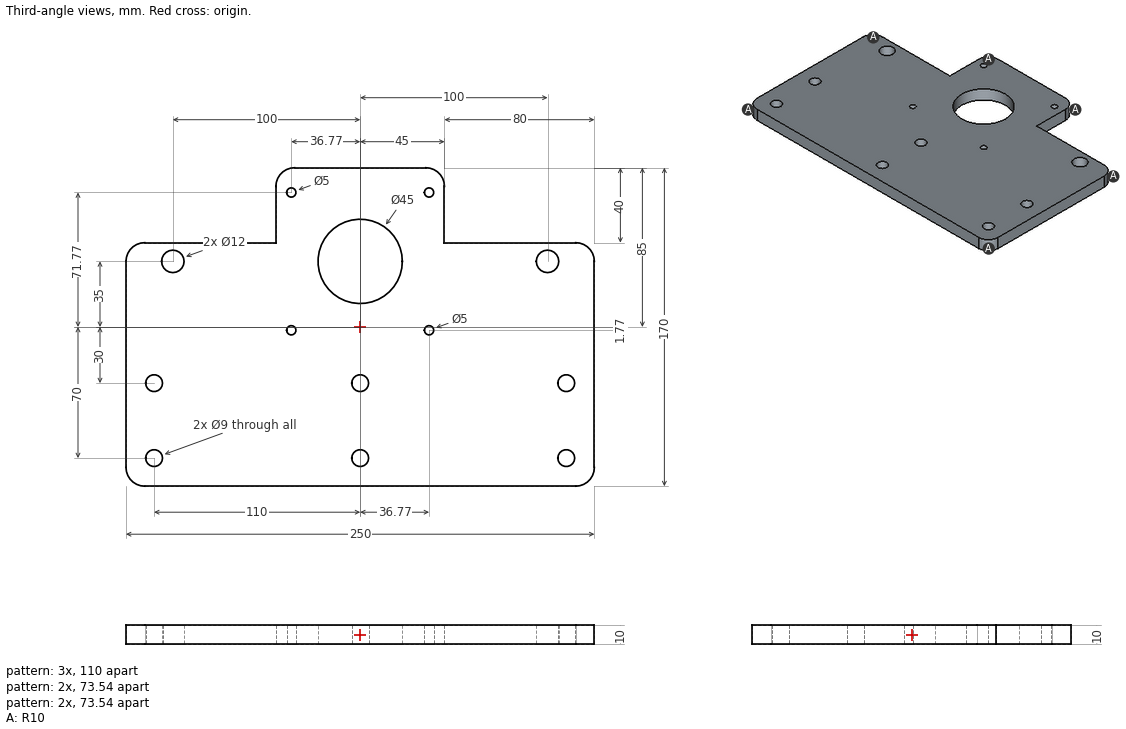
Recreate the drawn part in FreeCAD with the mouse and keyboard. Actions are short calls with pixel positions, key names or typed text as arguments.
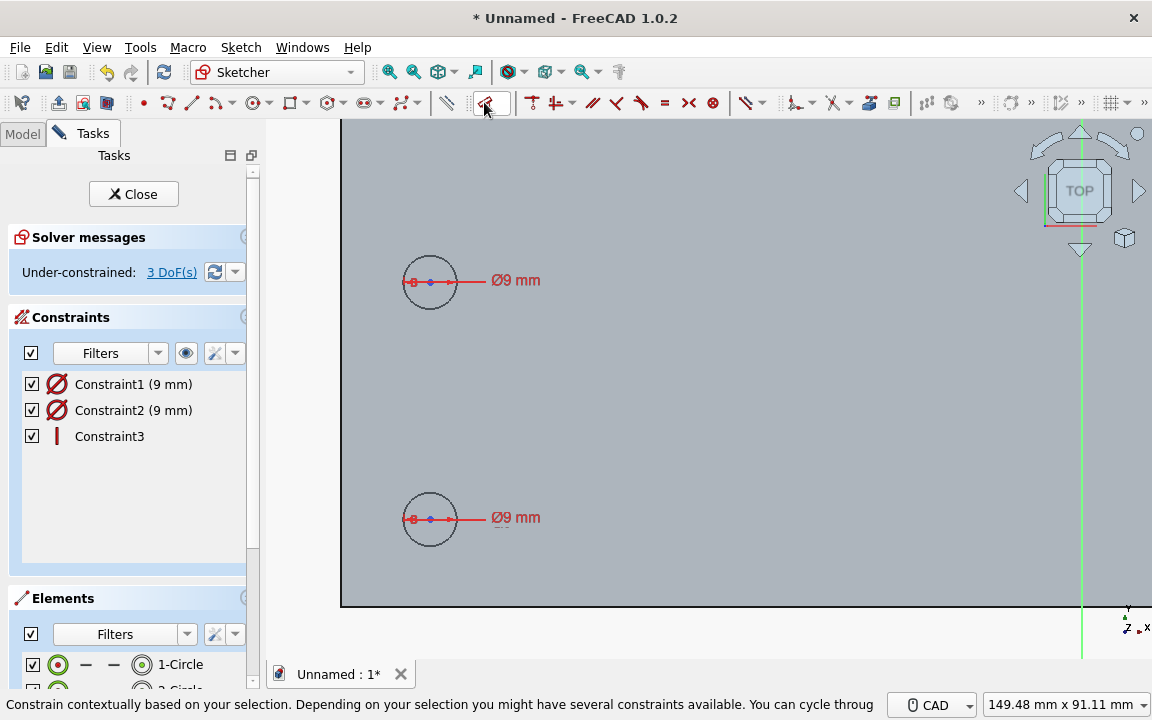
click(430, 520)
click(396, 333)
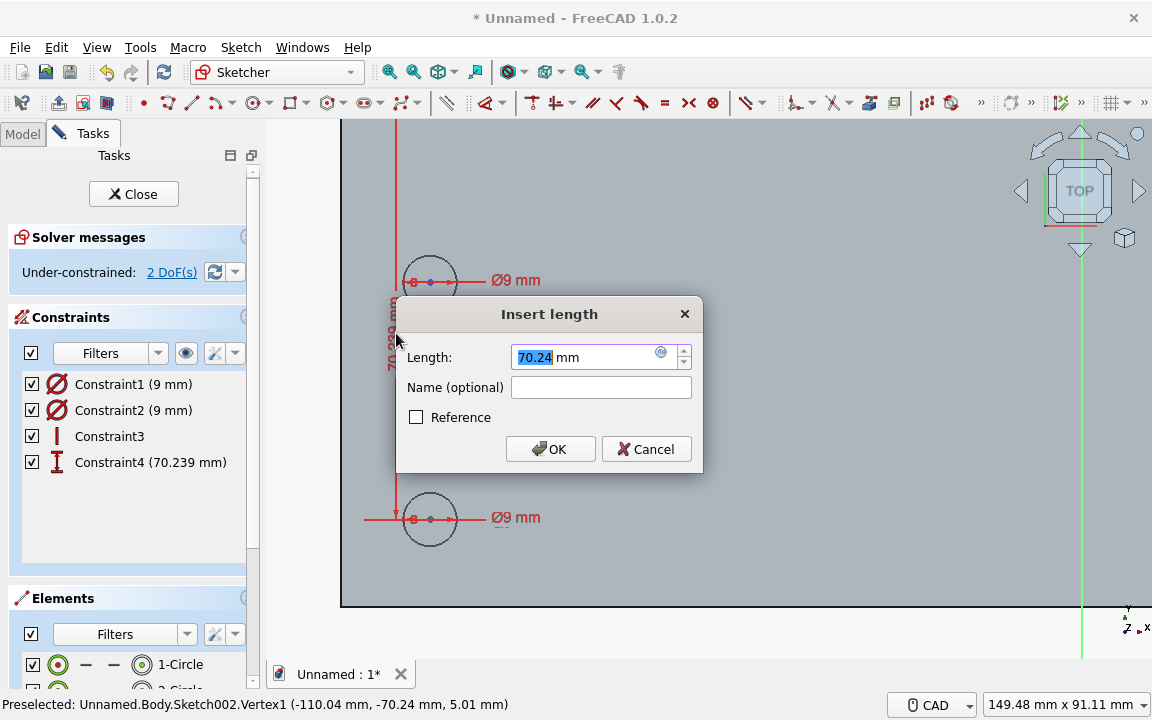
text(70)
key(Return)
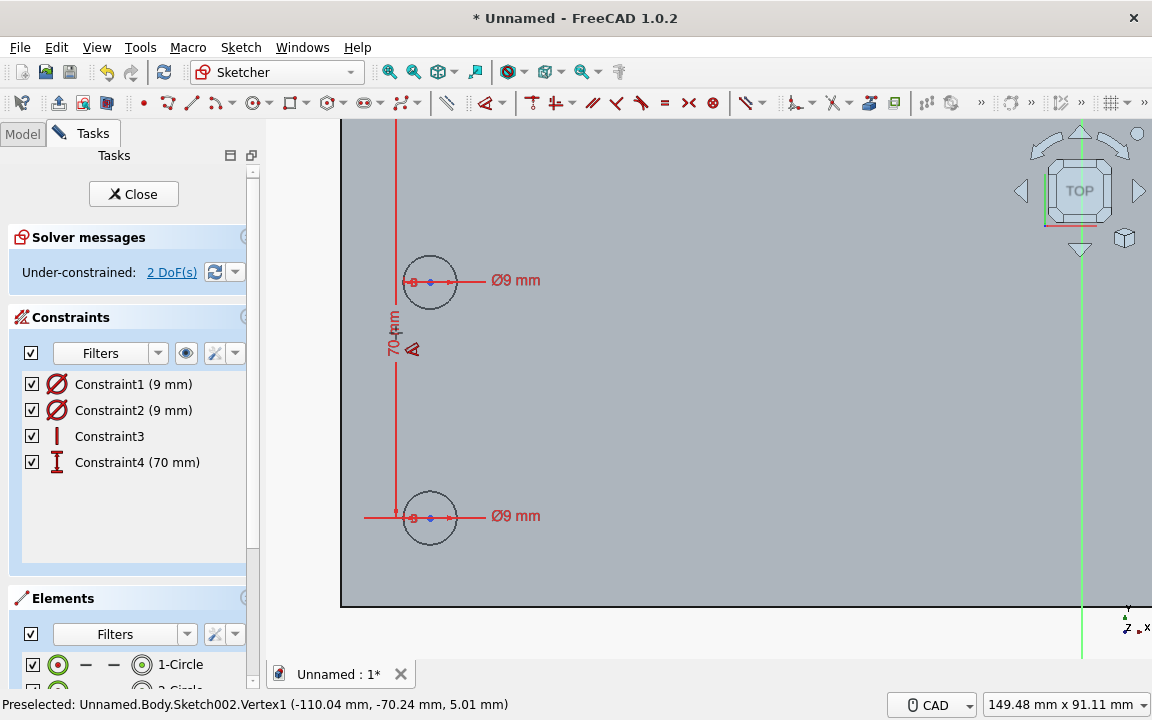
click(430, 282)
click(396, 215)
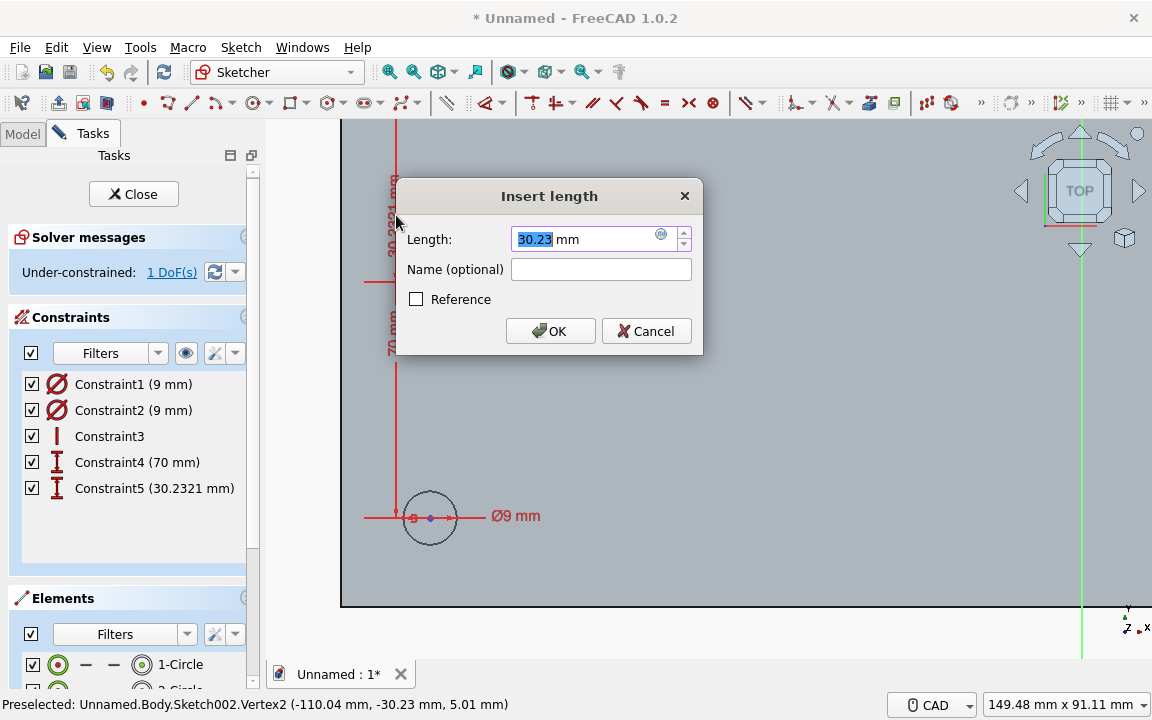
text(30)
key(Return)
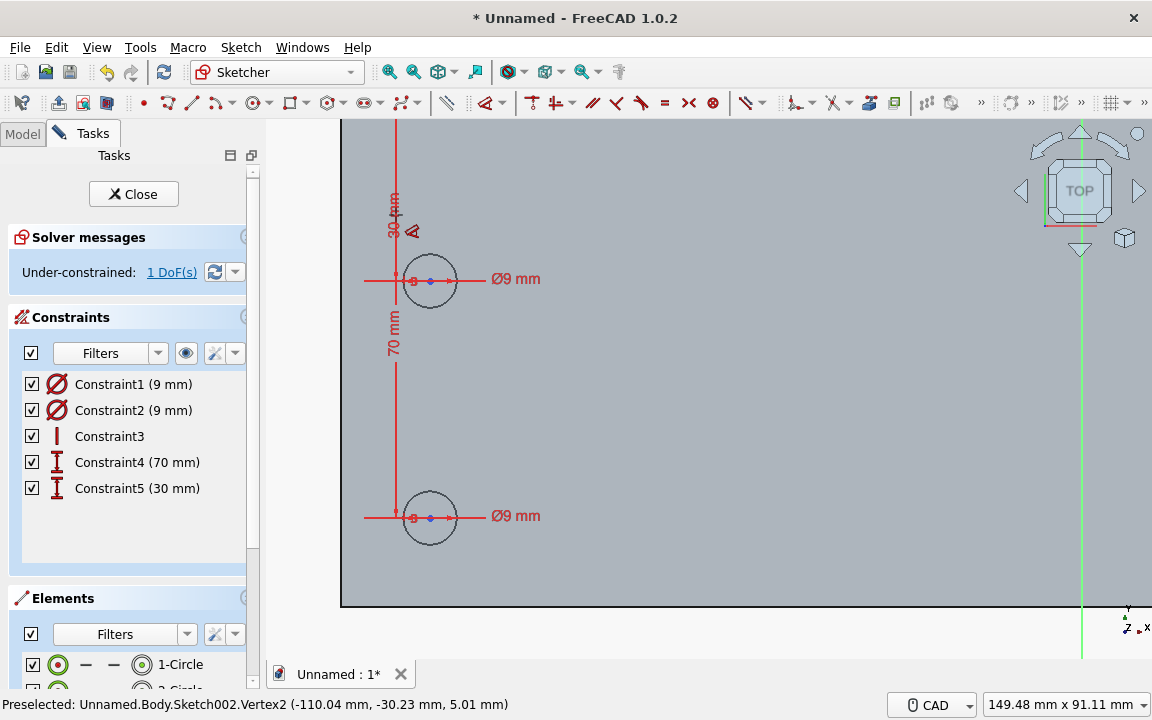
click(430, 518)
click(709, 552)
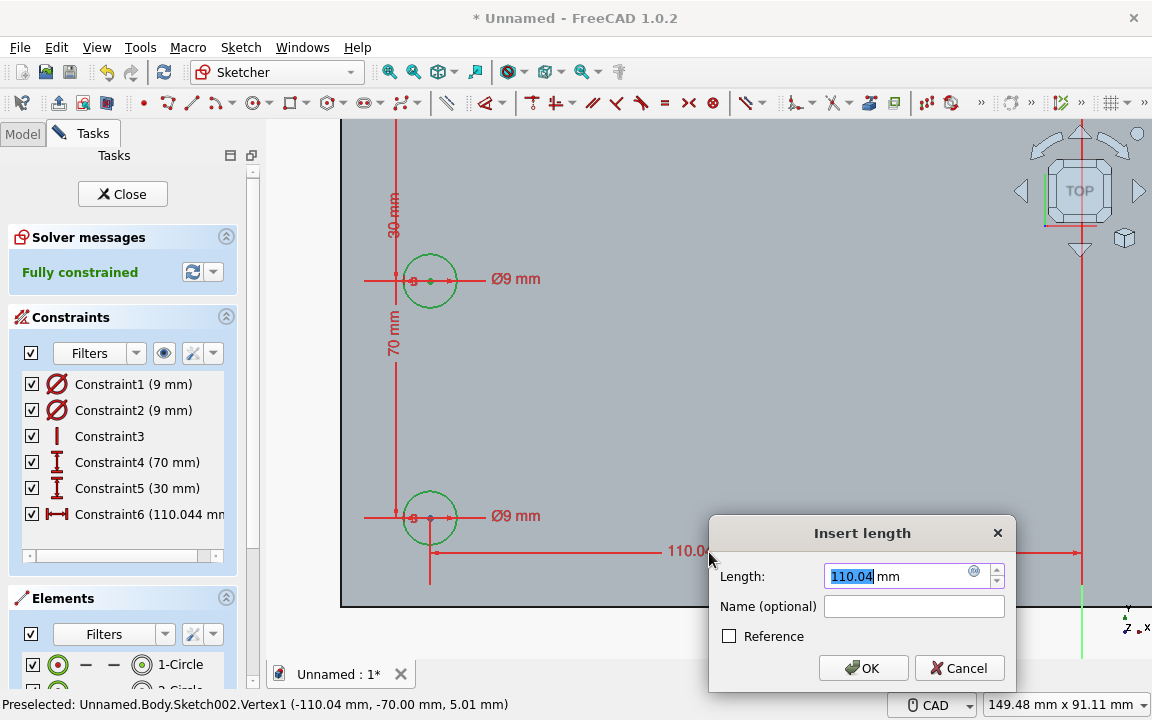
text(110)
key(Return)
key(Escape)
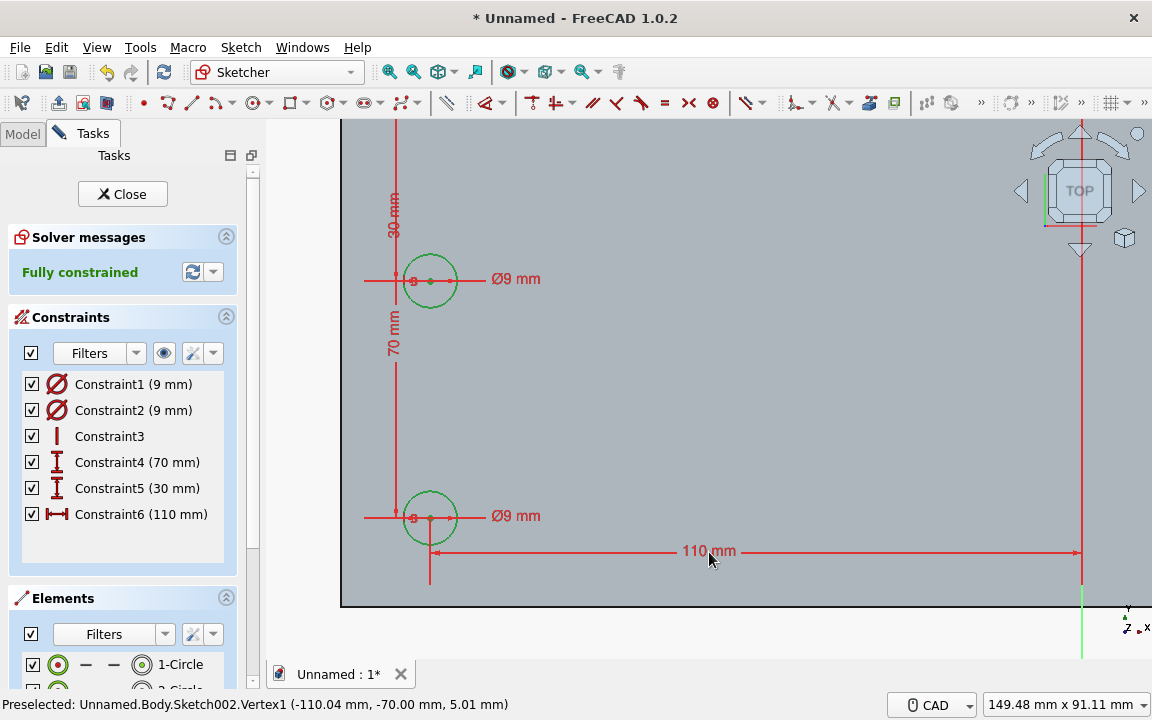
click(123, 194)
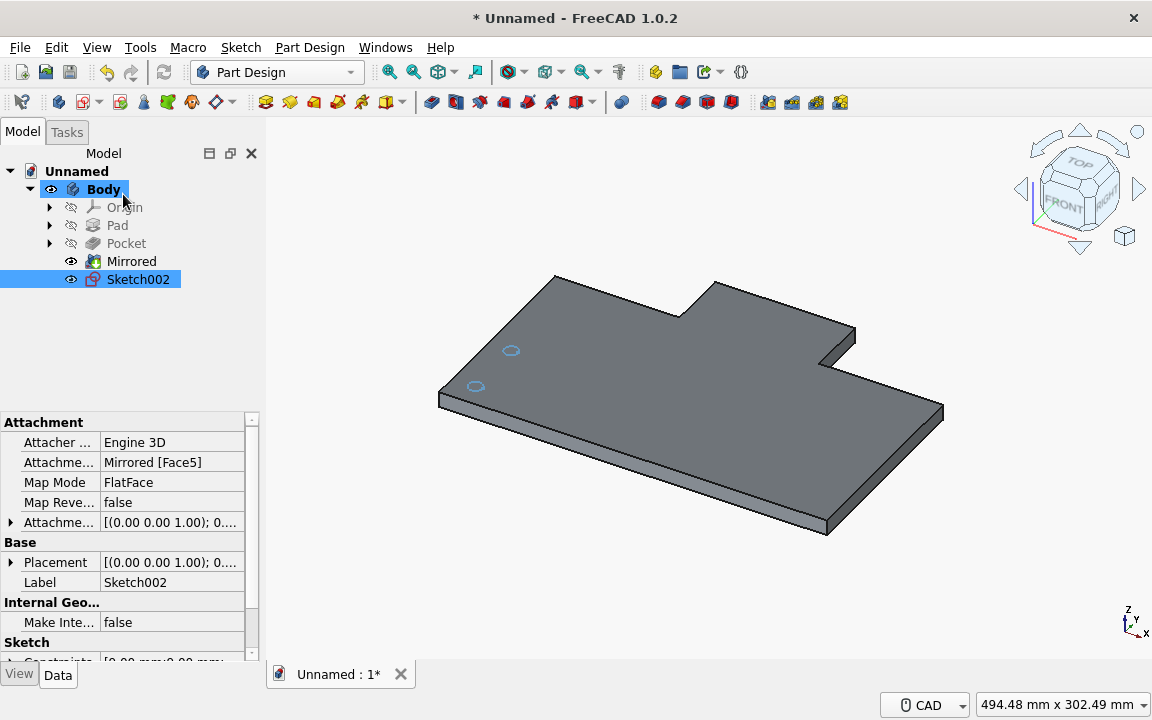
click(456, 102)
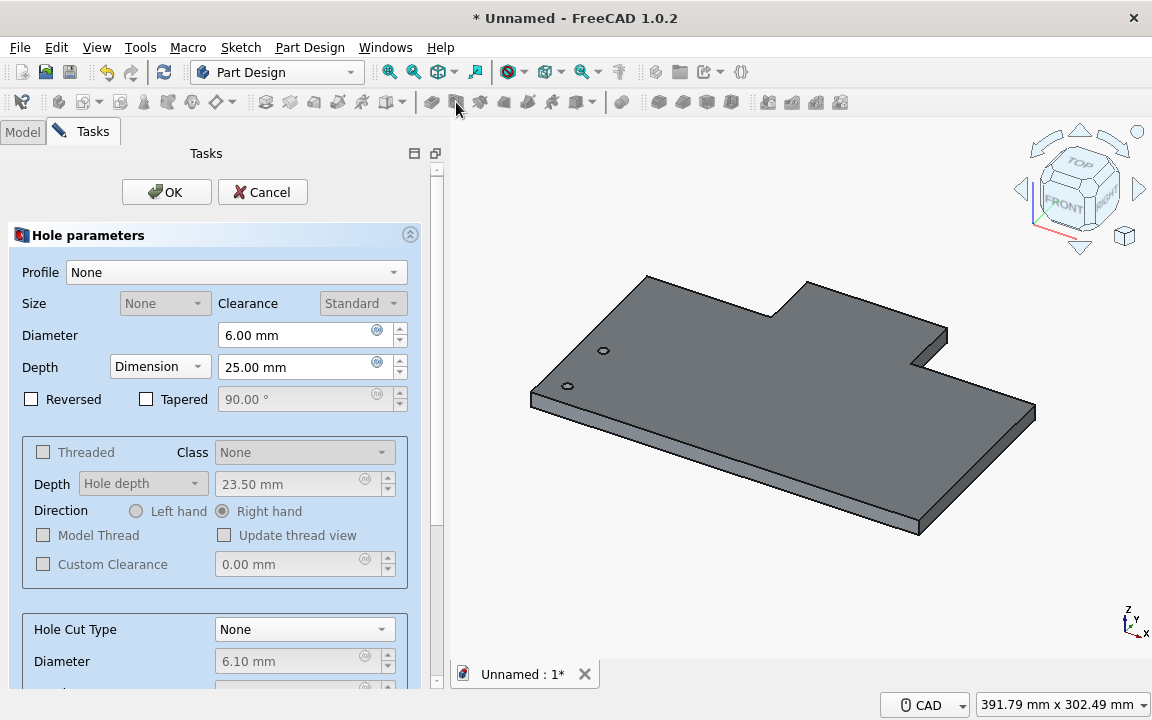
triple_click(305, 335)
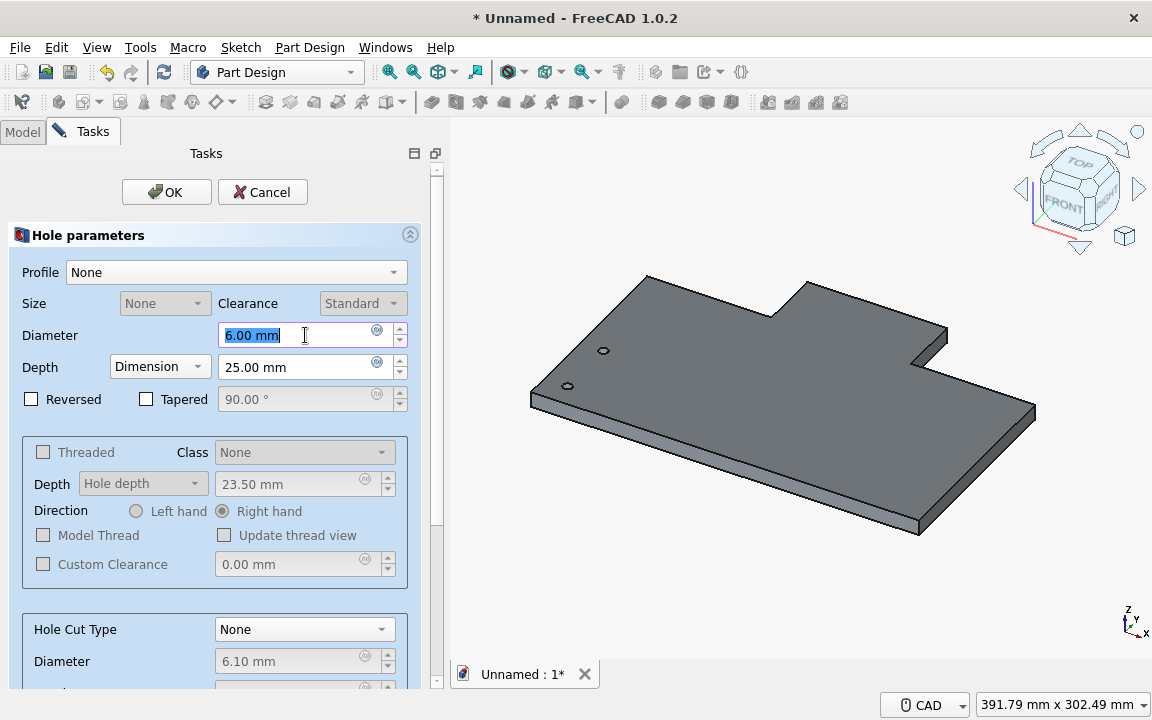
text(9)
key(Tab)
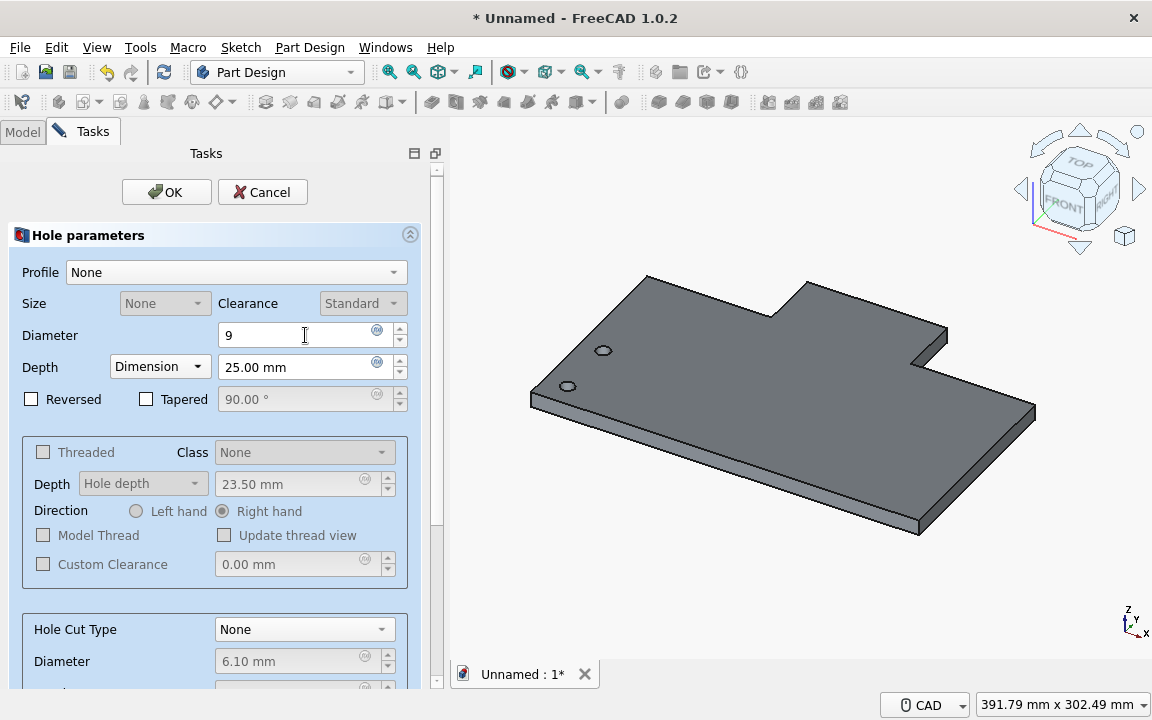
click(161, 366)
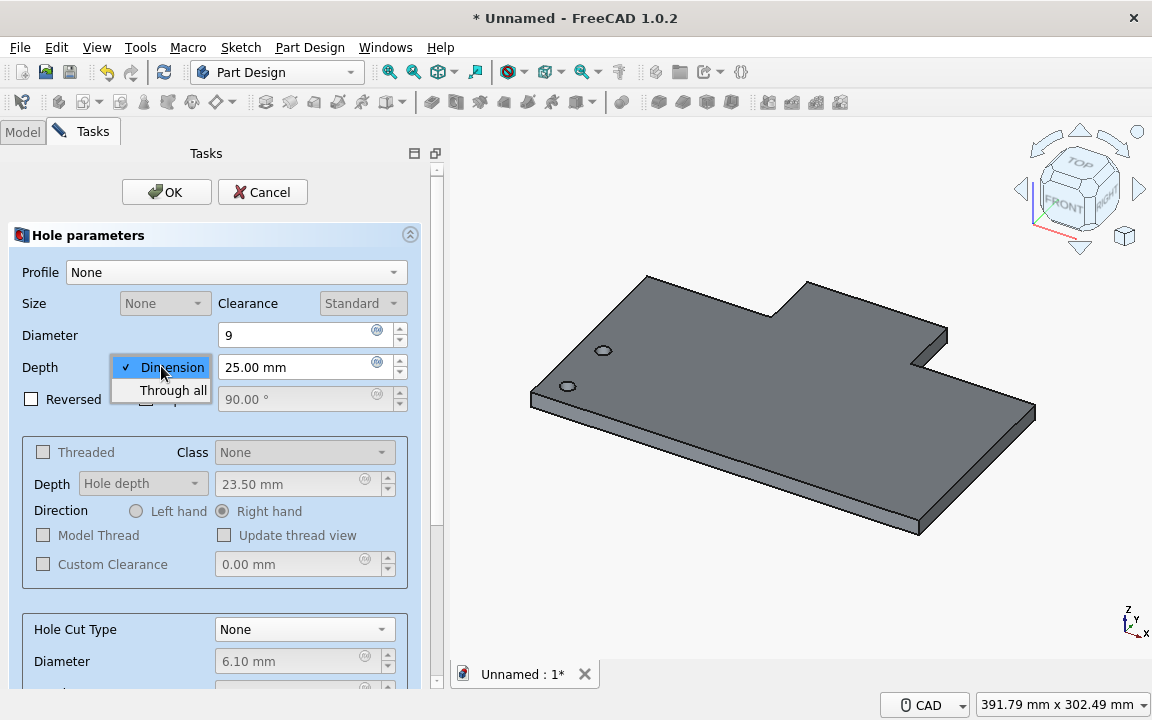
click(160, 390)